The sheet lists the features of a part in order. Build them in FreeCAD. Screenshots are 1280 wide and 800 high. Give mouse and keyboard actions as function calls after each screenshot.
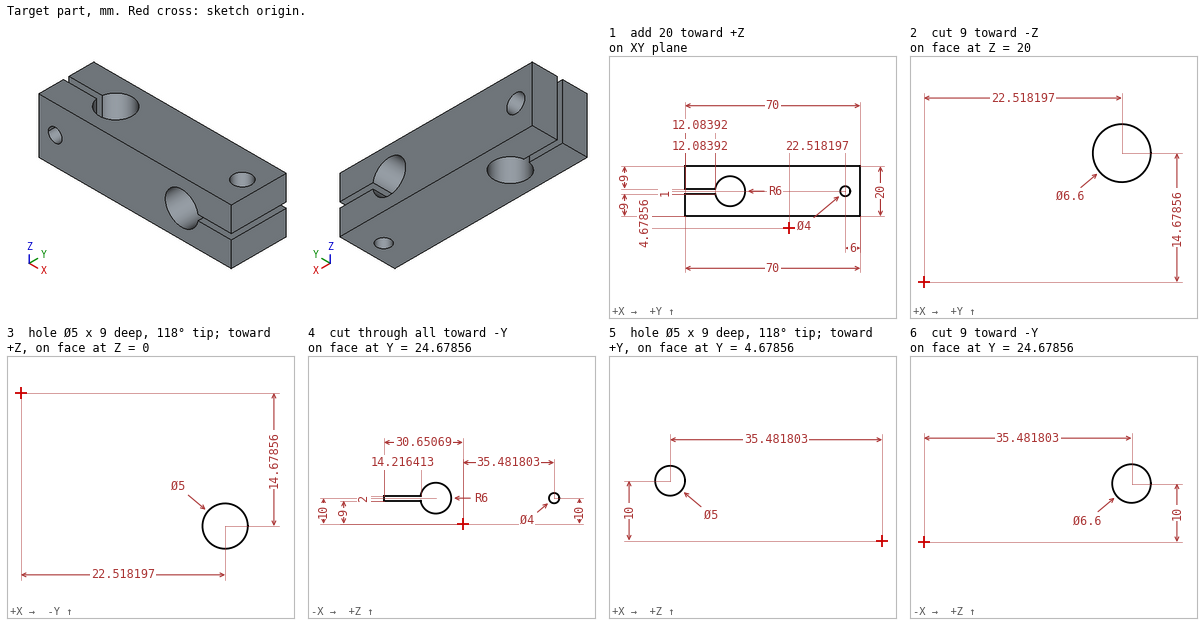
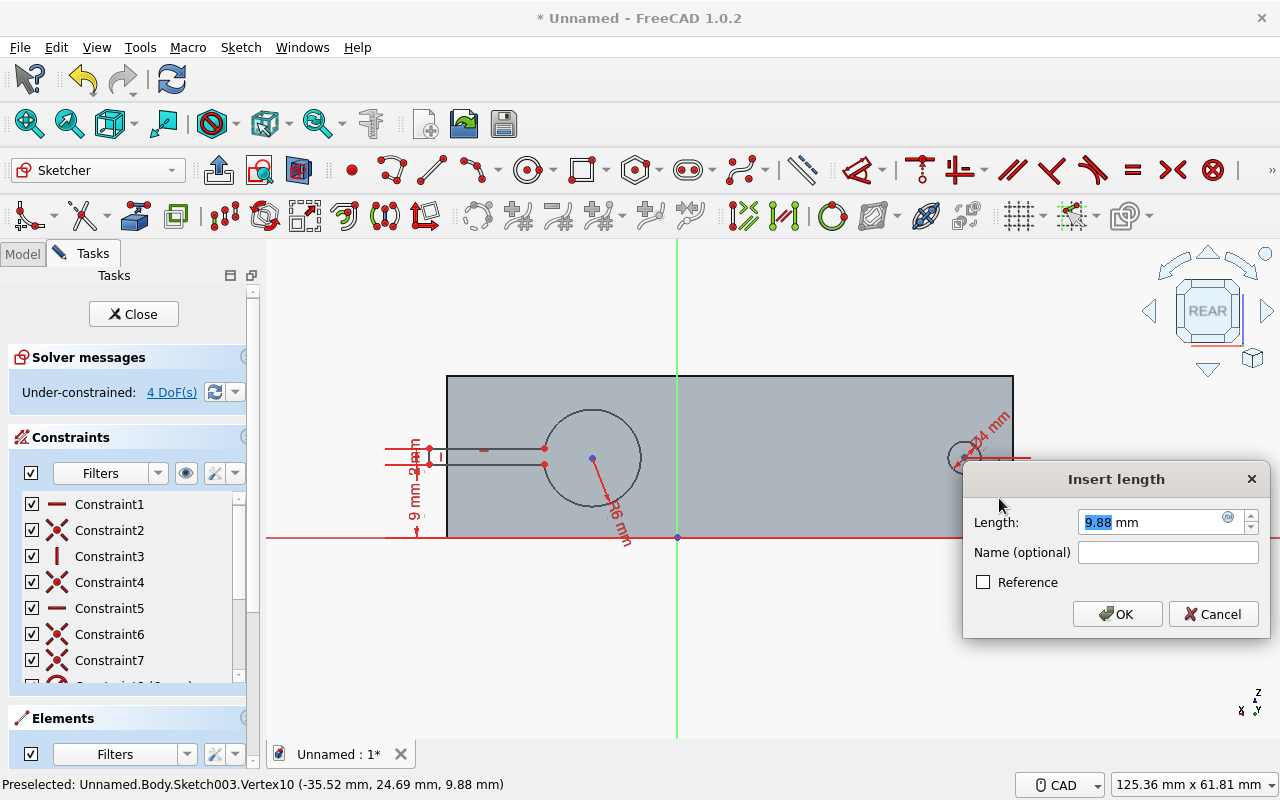
text(10)
key(Return)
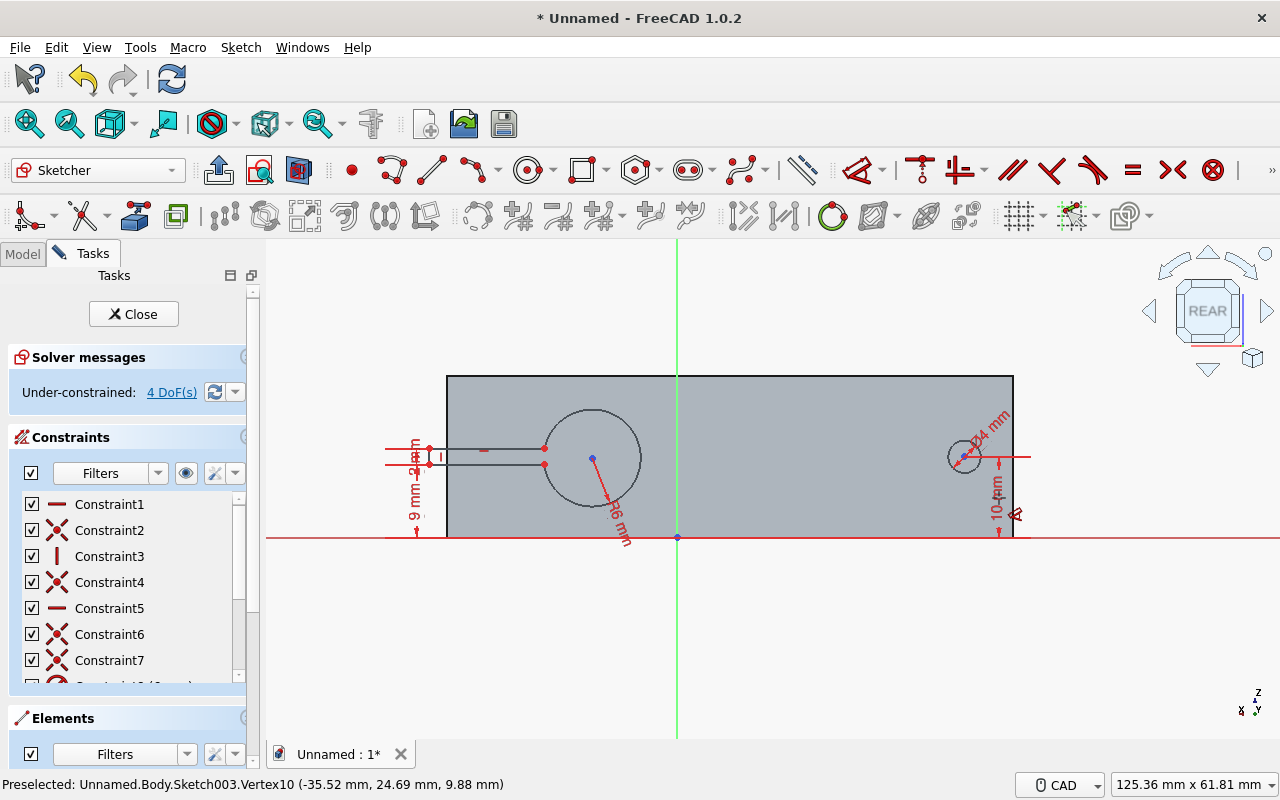
click(592, 458)
click(711, 498)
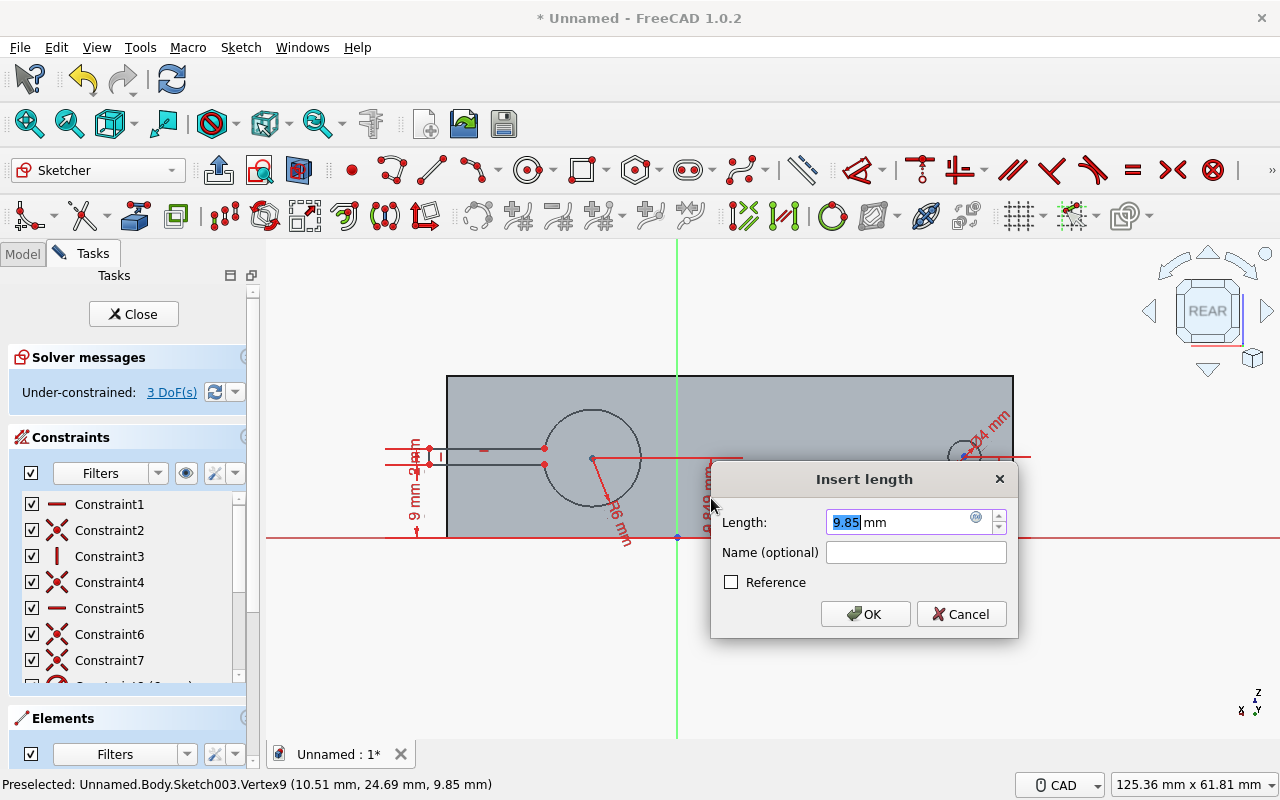
text(10)
key(Return)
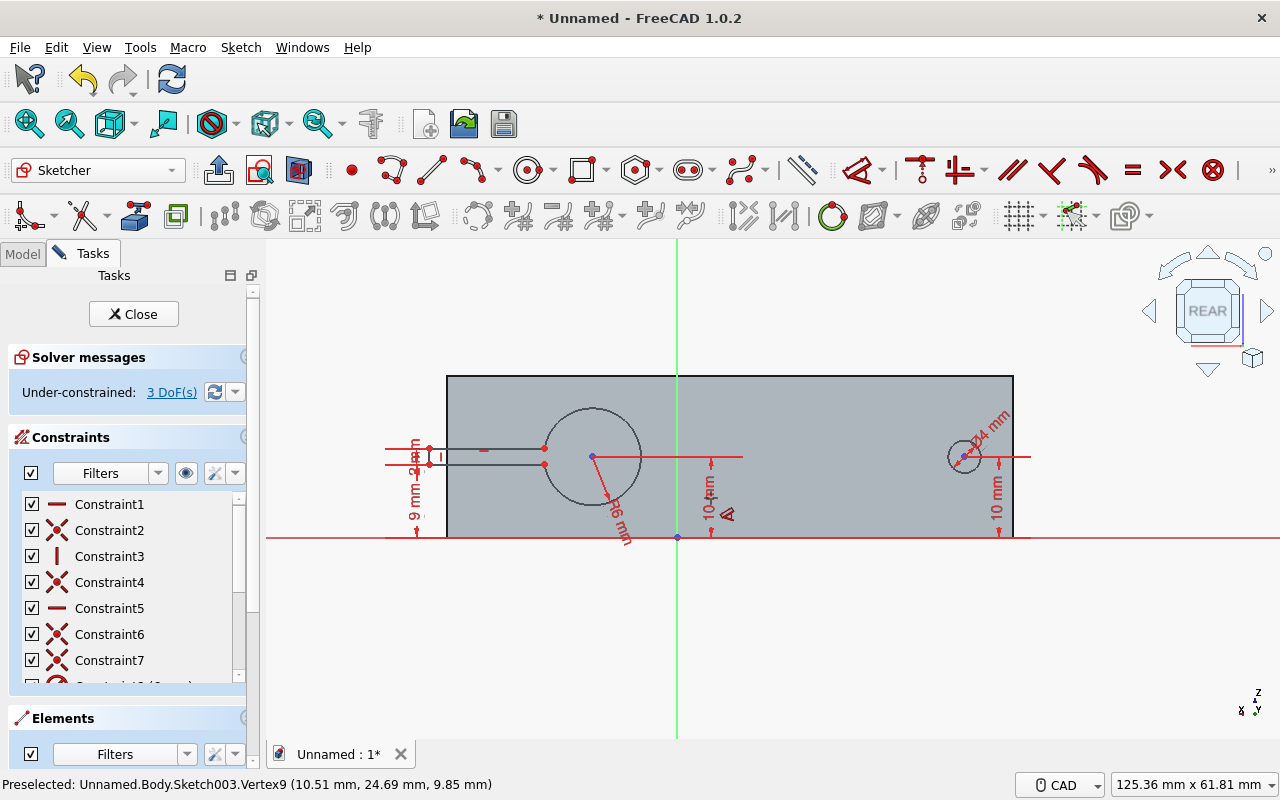
click(510, 449)
click(487, 415)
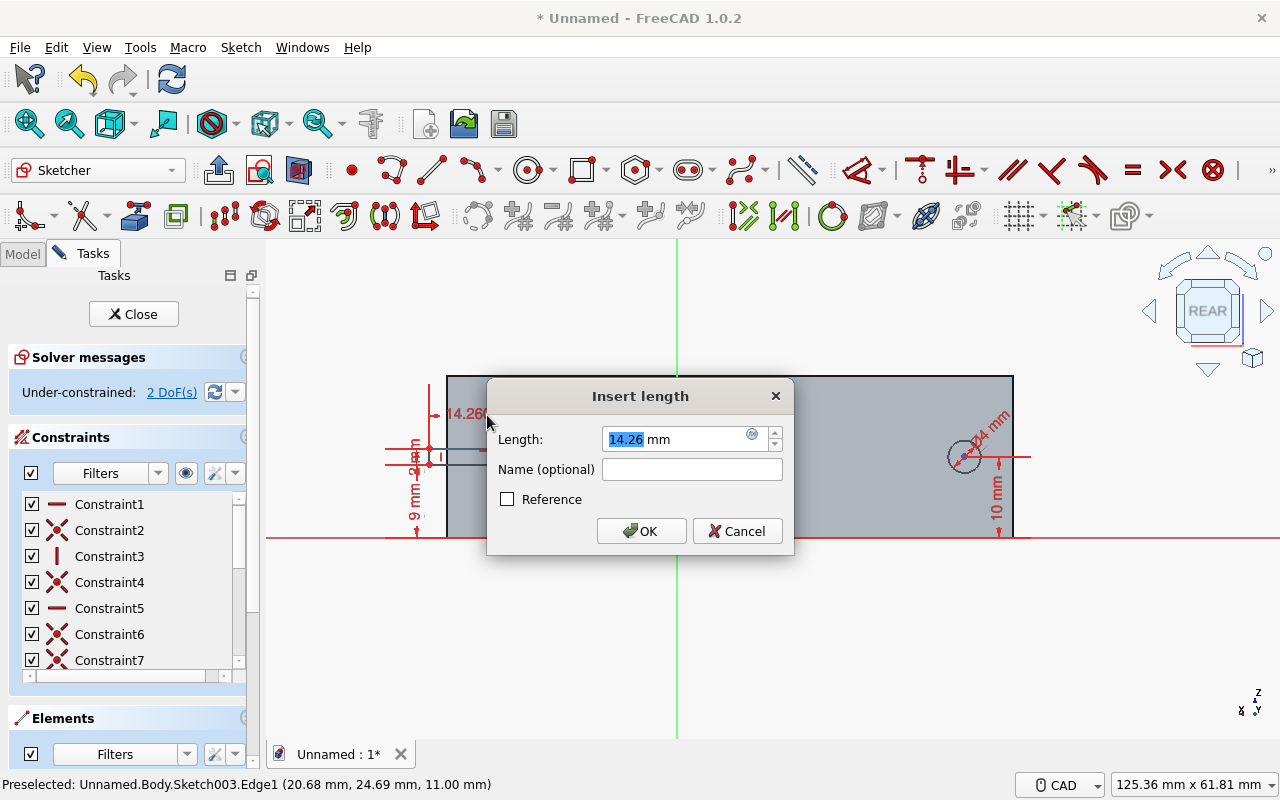
text(14.216413)
key(Return)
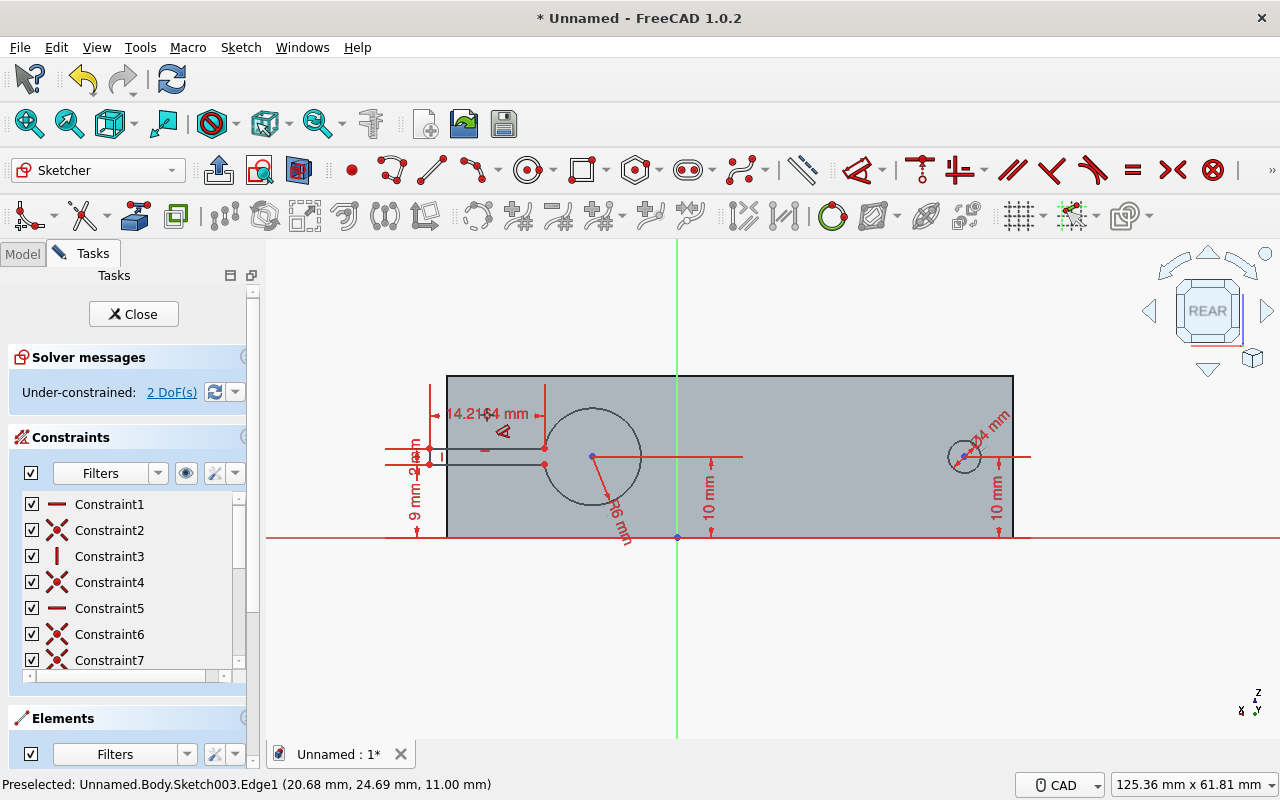
click(430, 449)
click(553, 572)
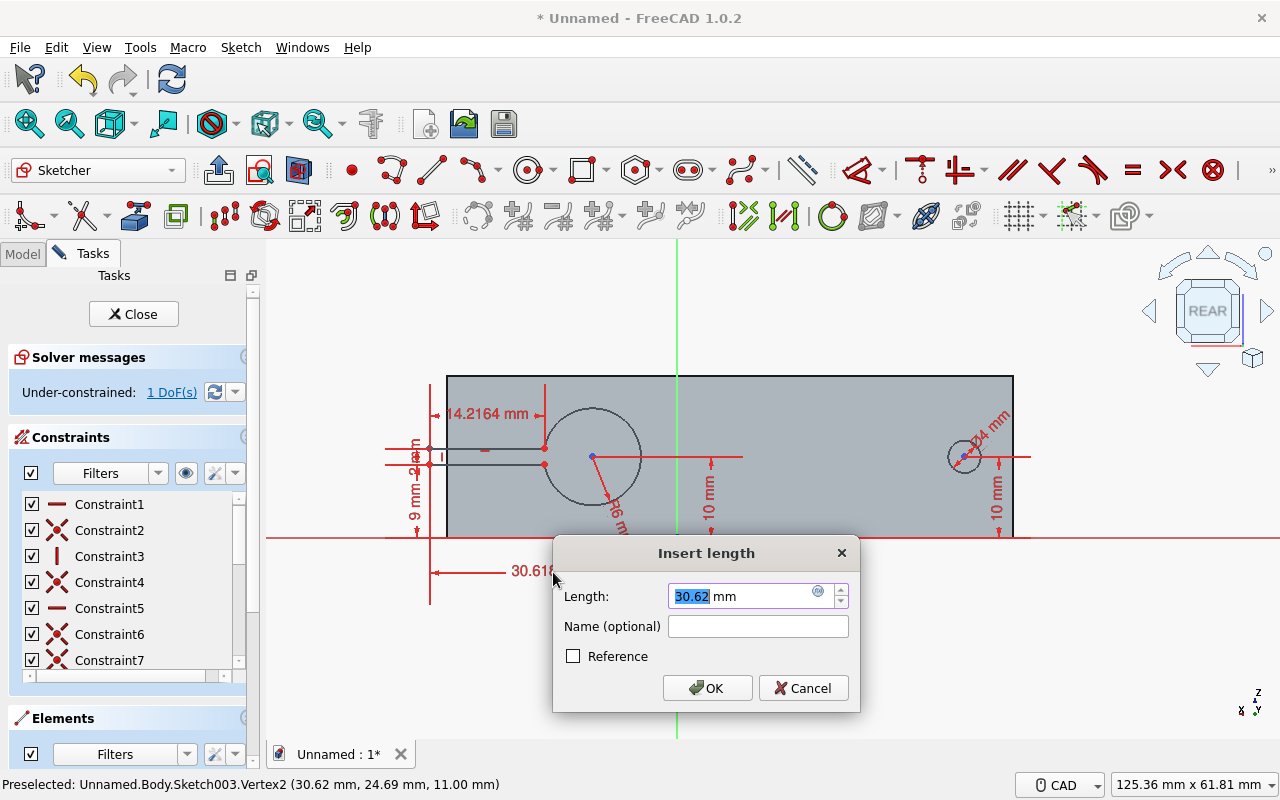
text(30.65069)
key(Return)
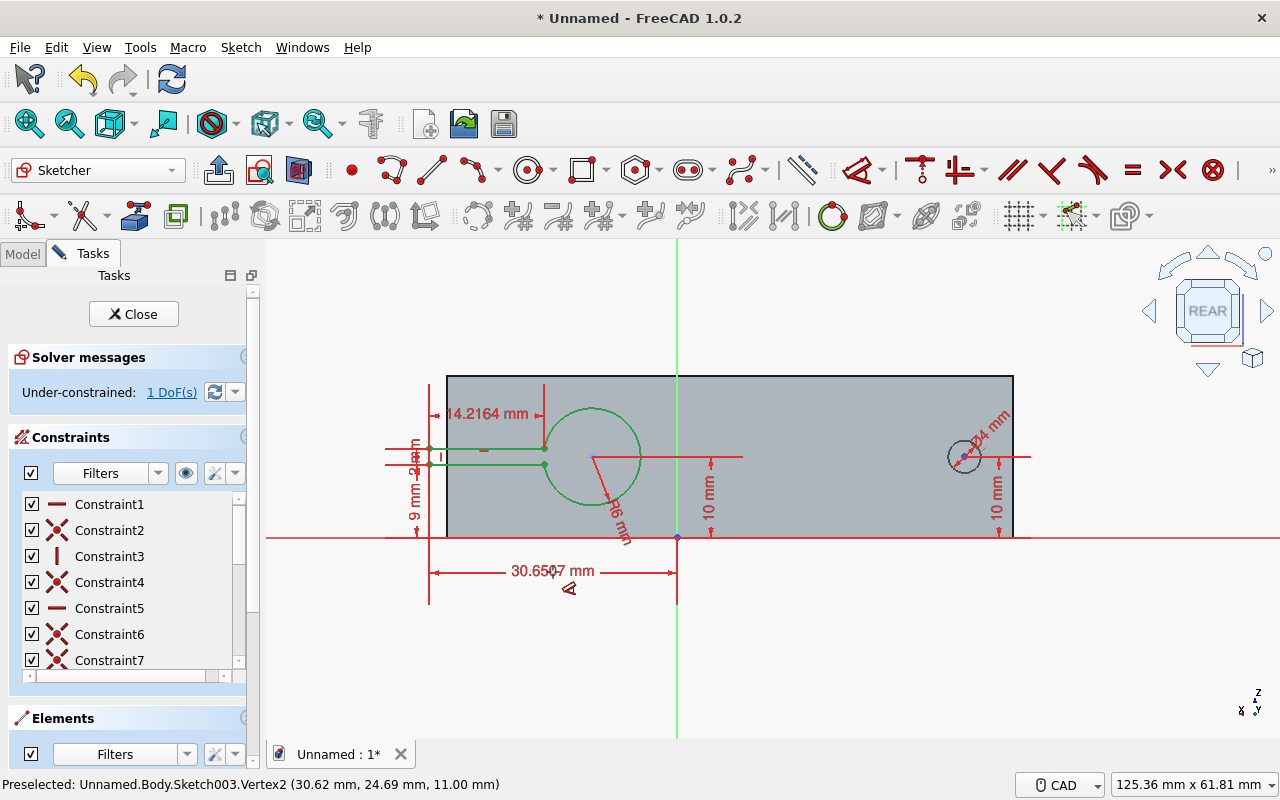
click(965, 457)
click(821, 572)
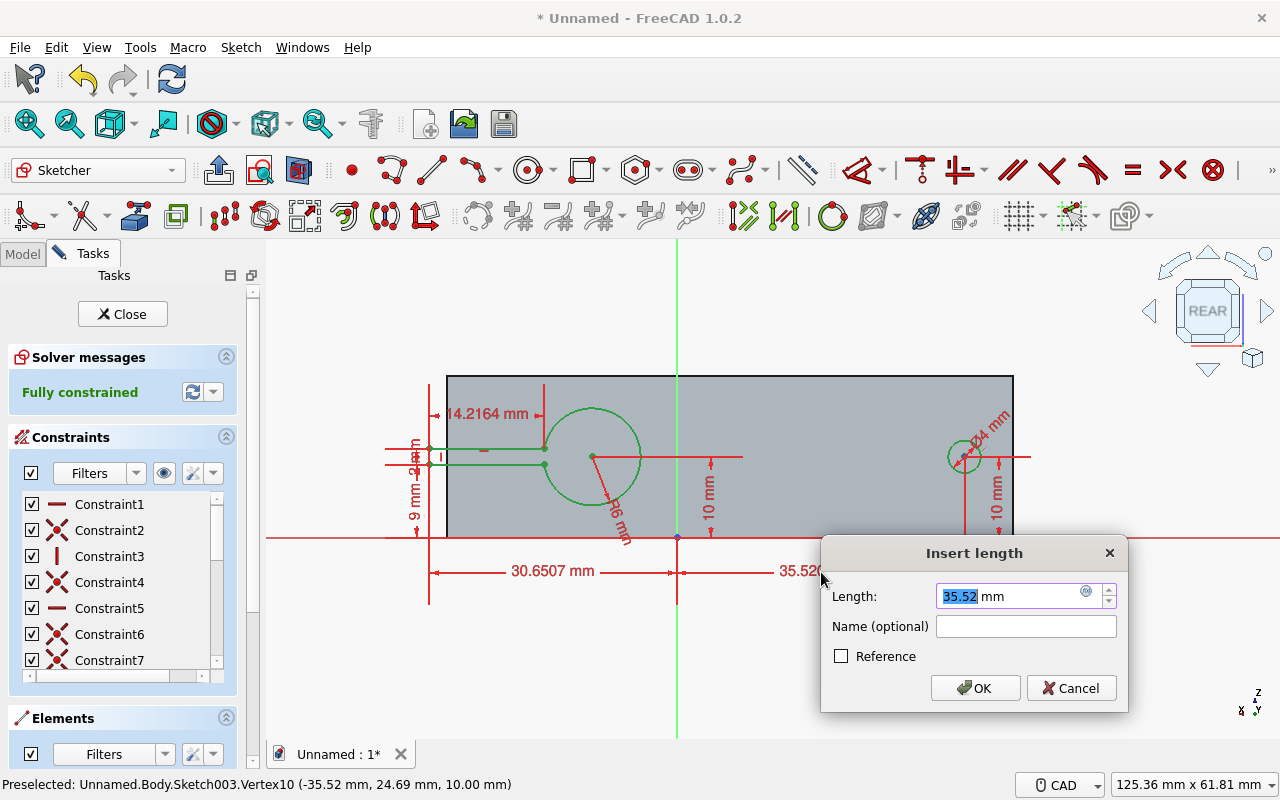
text(35.481803)
key(Return)
key(Escape)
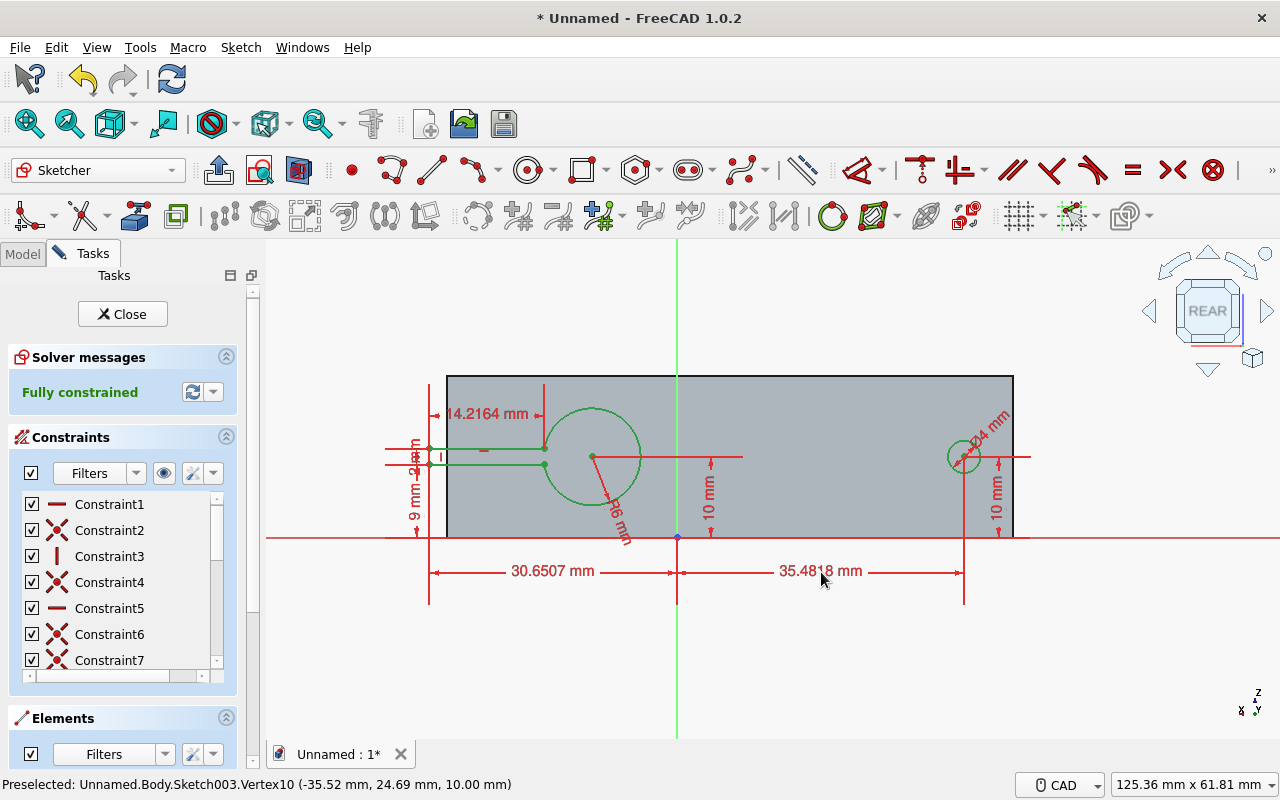
click(123, 314)